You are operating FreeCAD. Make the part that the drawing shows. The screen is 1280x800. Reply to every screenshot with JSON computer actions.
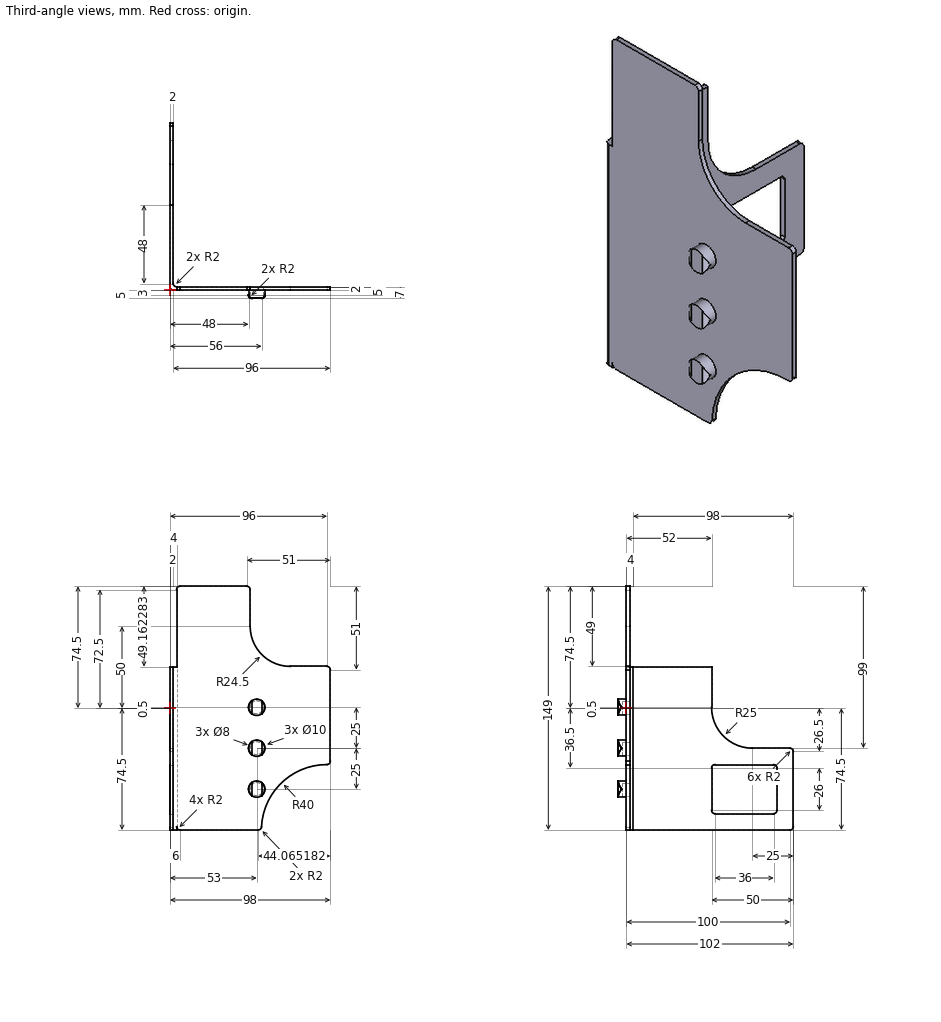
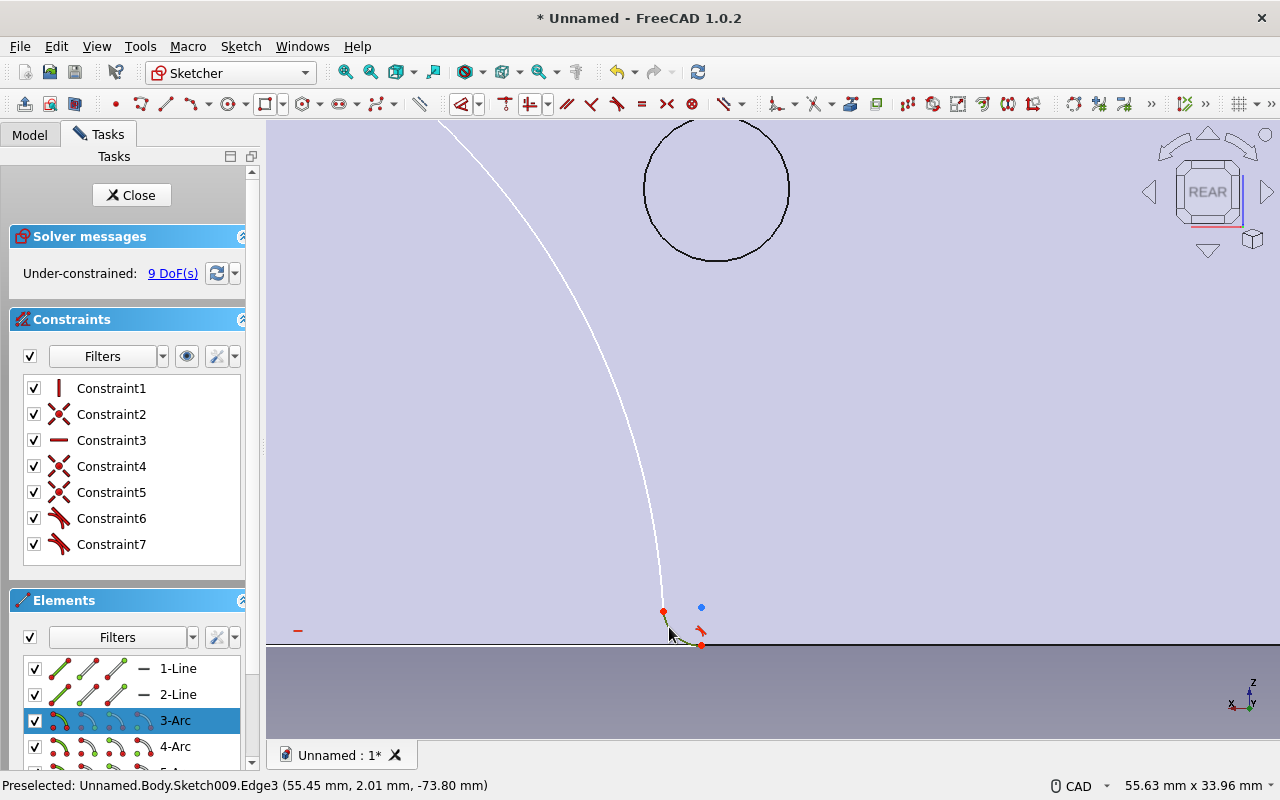
{"action": "left_click", "coordinate": [572, 294]}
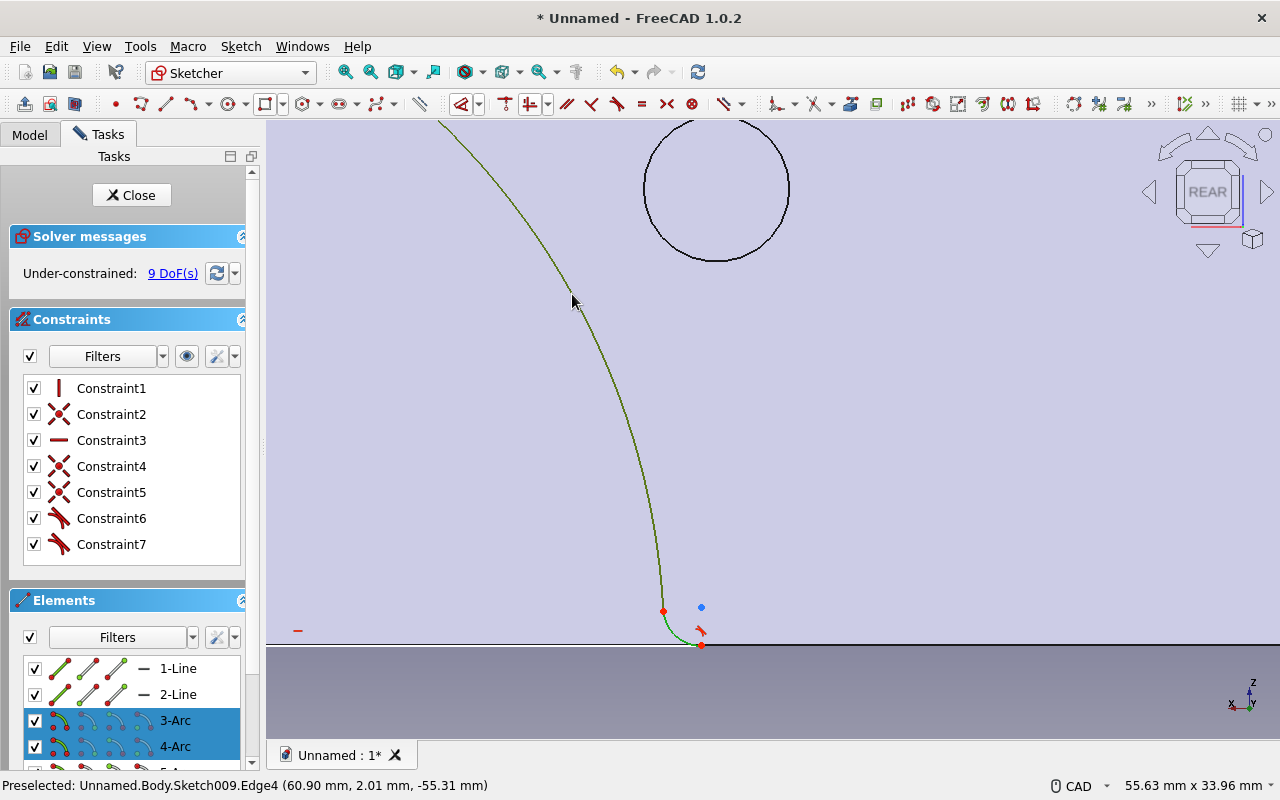
{"action": "left_click", "coordinate": [617, 104]}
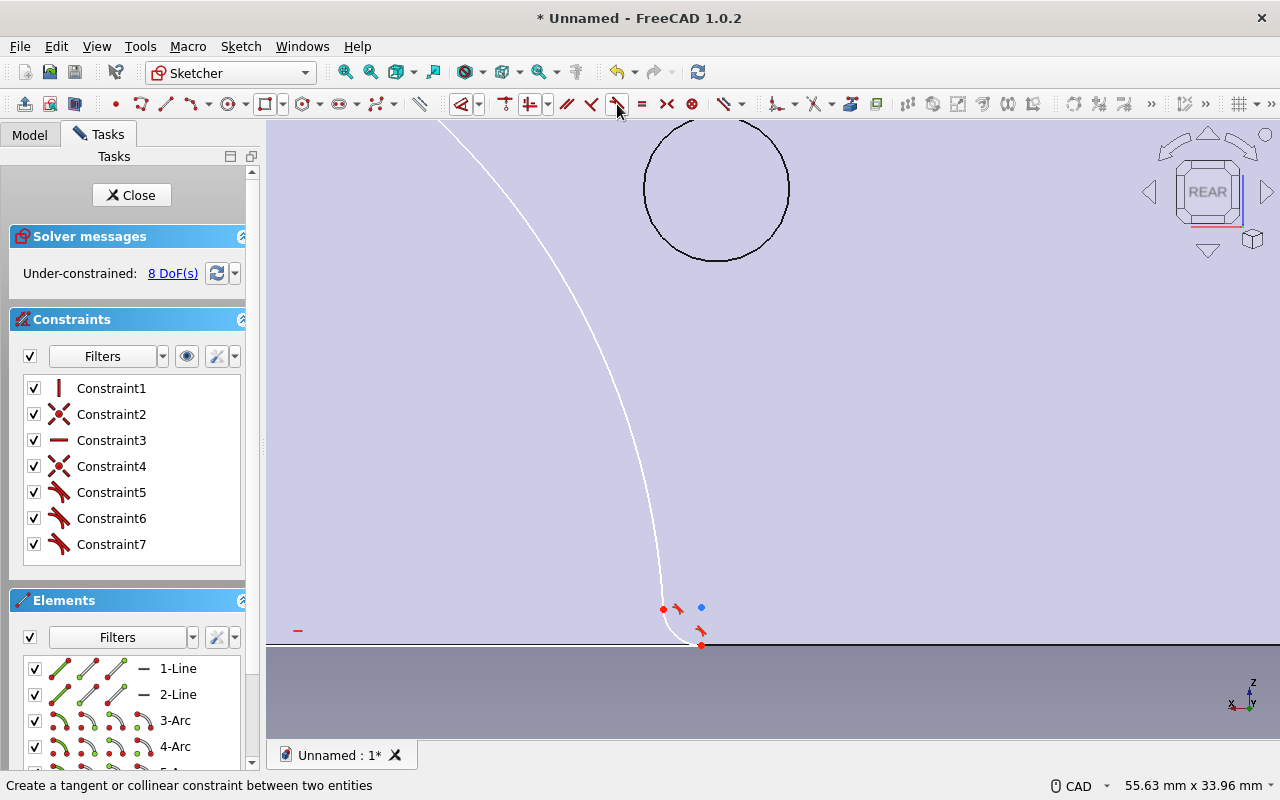
{"action": "left_click", "coordinate": [572, 293]}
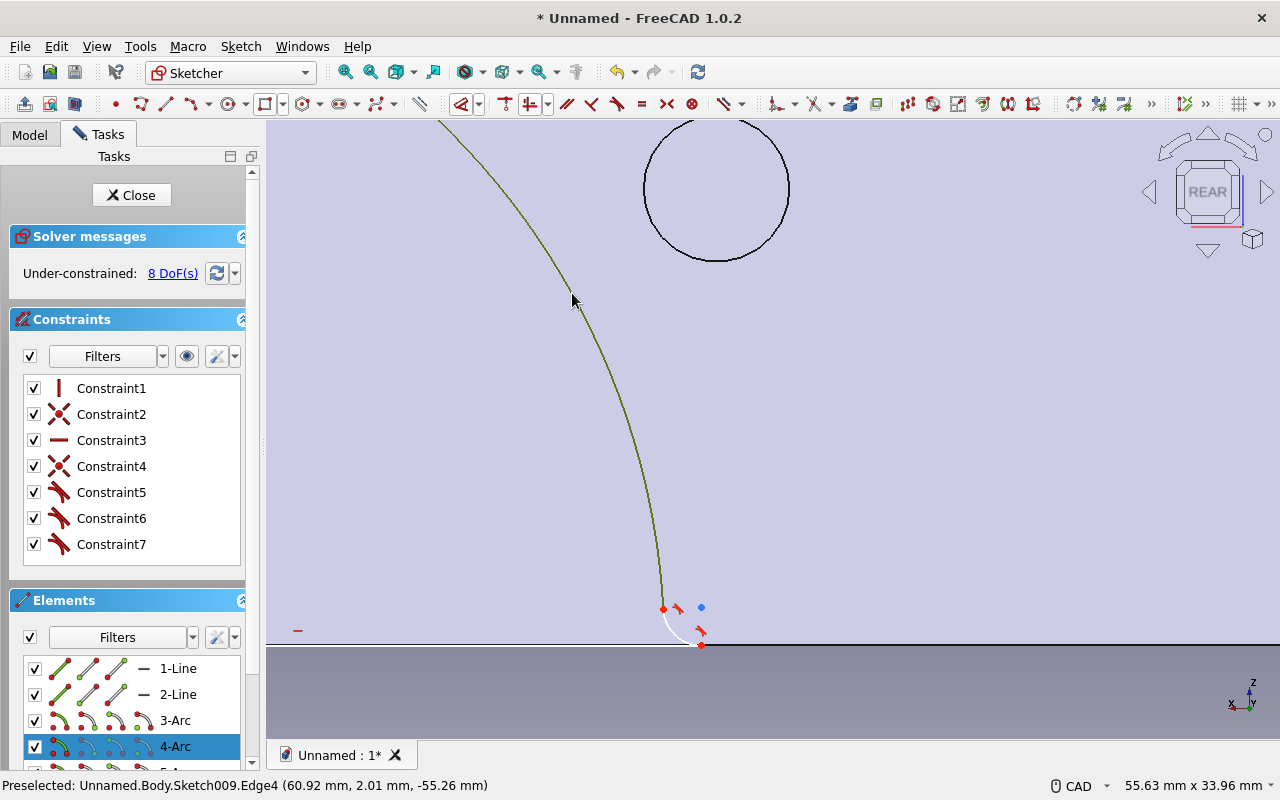
{"action": "scroll", "coordinate": [668, 629], "scroll_direction": "down", "scroll_amount": 6}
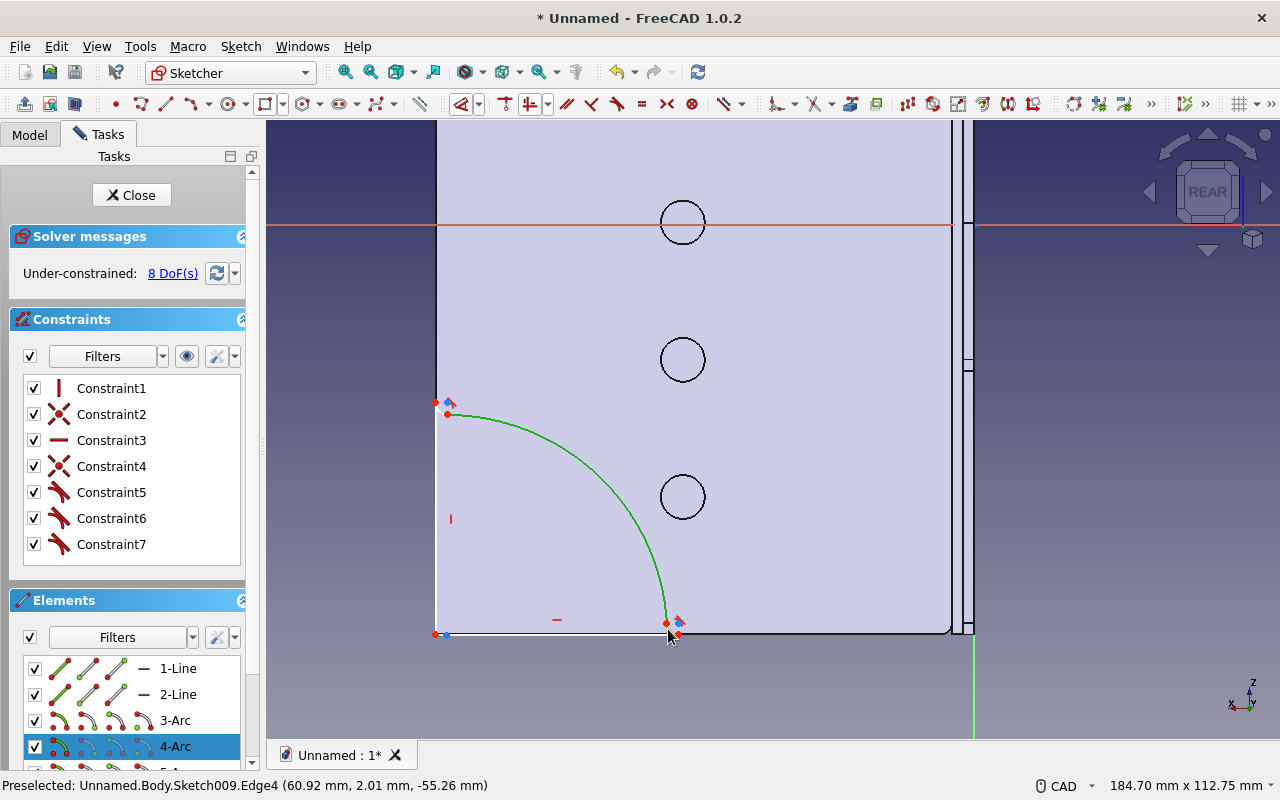
{"action": "scroll", "coordinate": [442, 413], "scroll_direction": "up", "scroll_amount": 5}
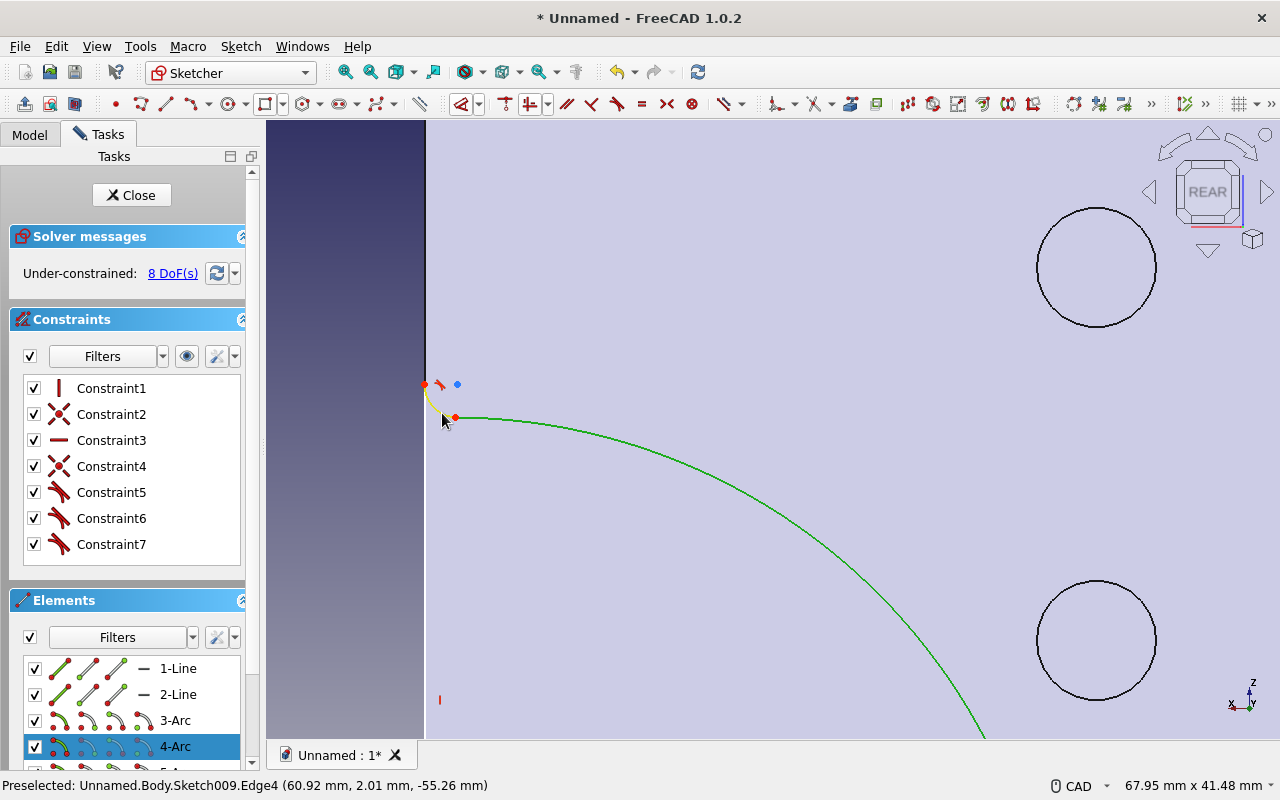
{"action": "left_click", "coordinate": [441, 413]}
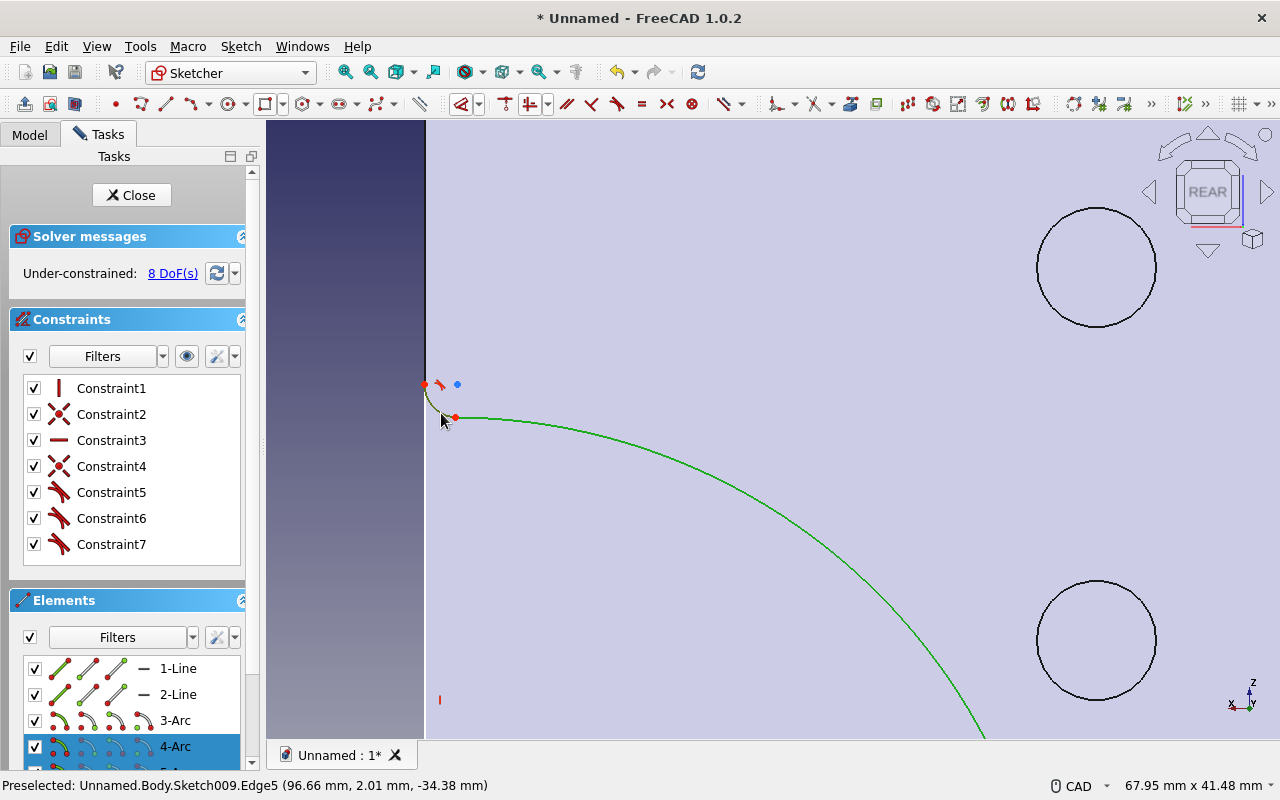
{"action": "left_click", "coordinate": [617, 104]}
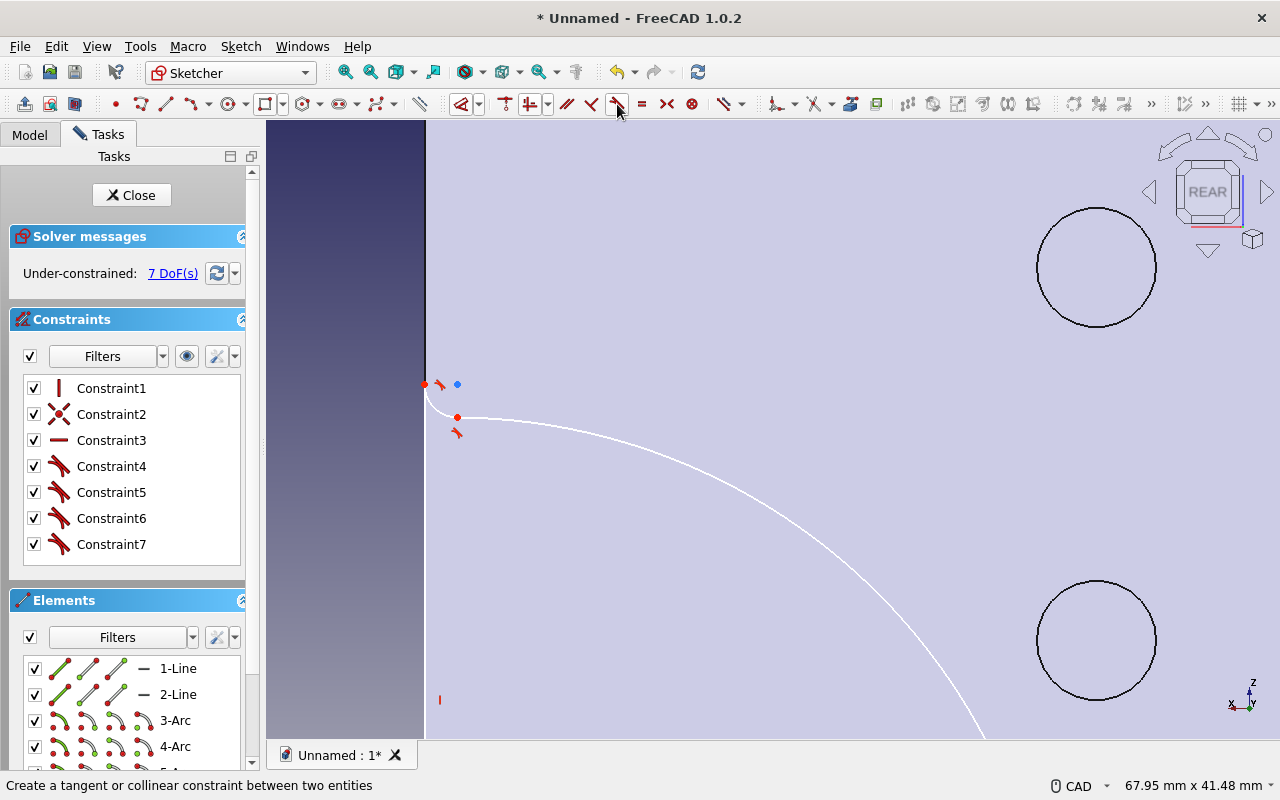
{"action": "scroll", "coordinate": [442, 413], "scroll_direction": "down", "scroll_amount": 5}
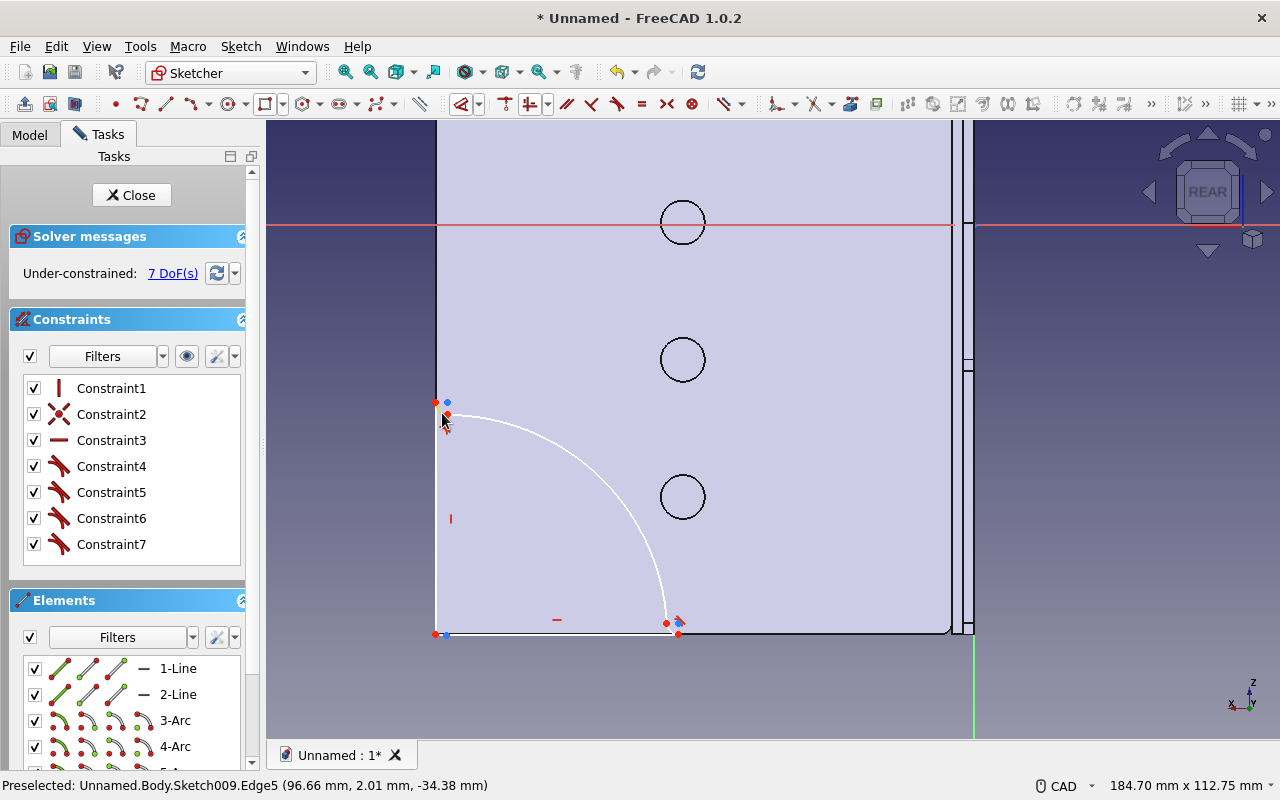
{"action": "scroll", "coordinate": [668, 629], "scroll_direction": "up", "scroll_amount": 5}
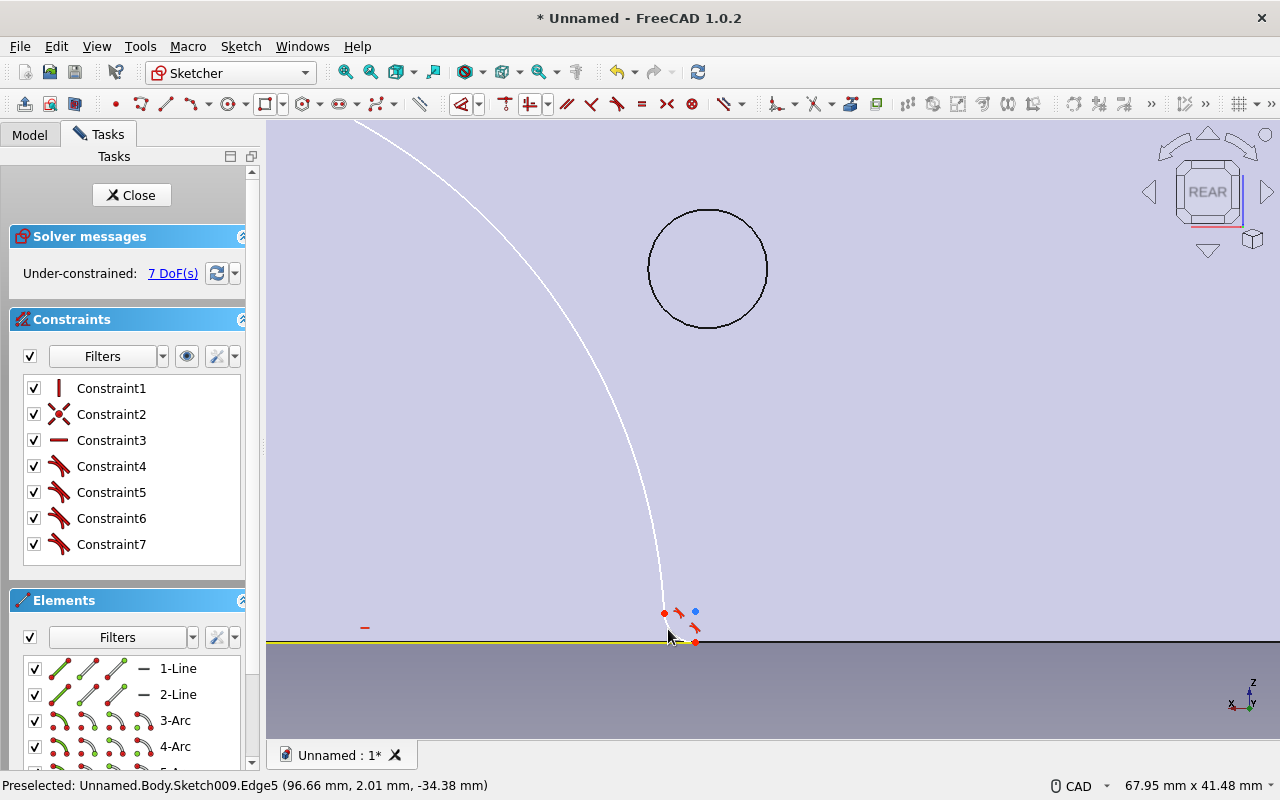
{"action": "left_click", "coordinate": [668, 627]}